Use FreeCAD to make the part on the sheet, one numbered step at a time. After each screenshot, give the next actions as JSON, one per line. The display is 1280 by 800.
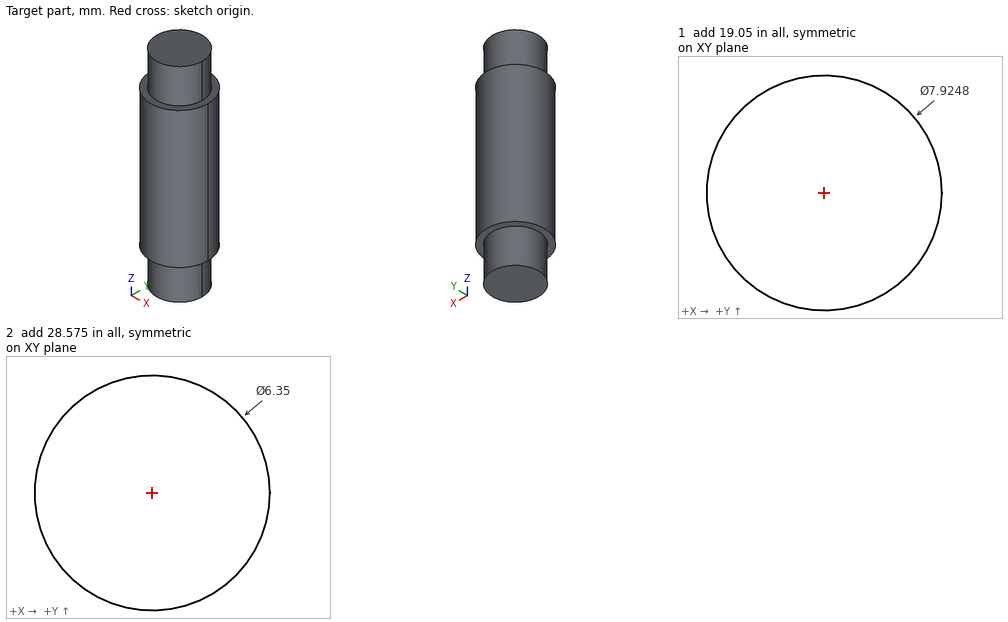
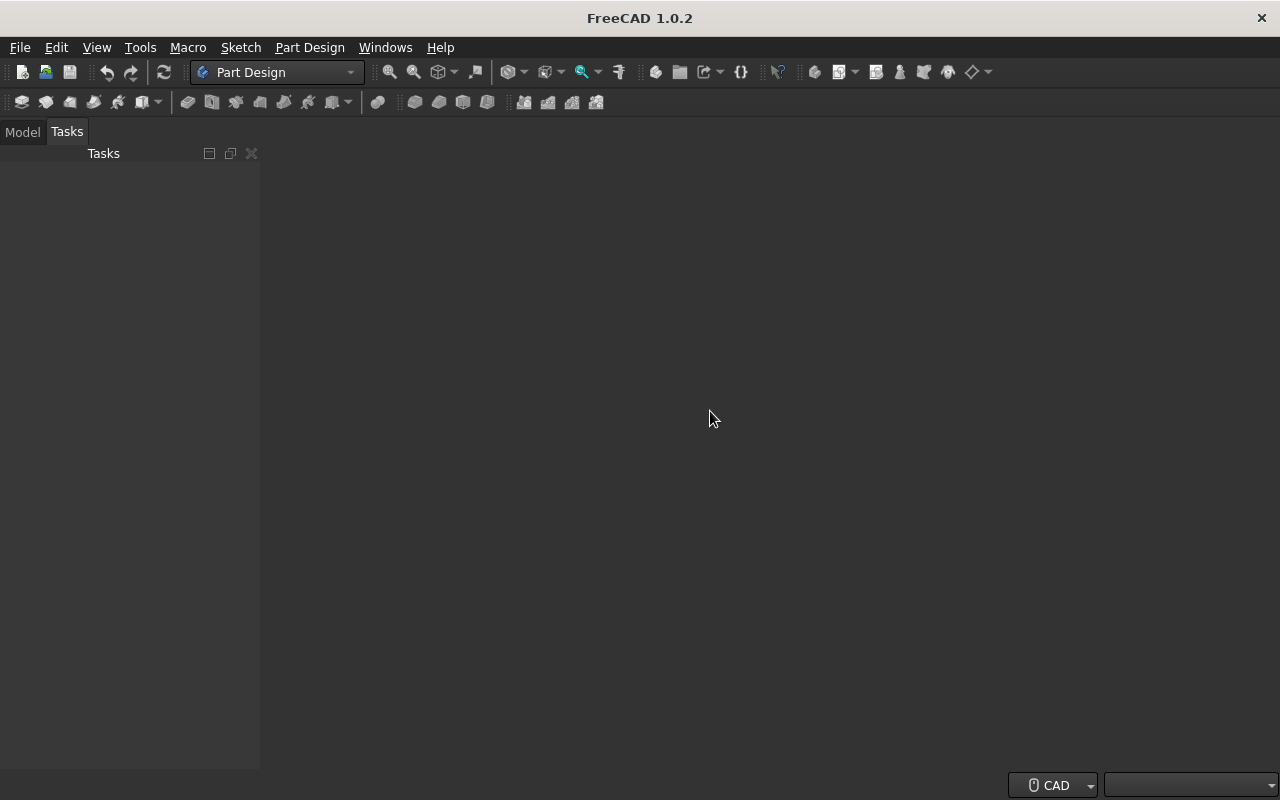
{"action": "left_click", "coordinate": [22, 72]}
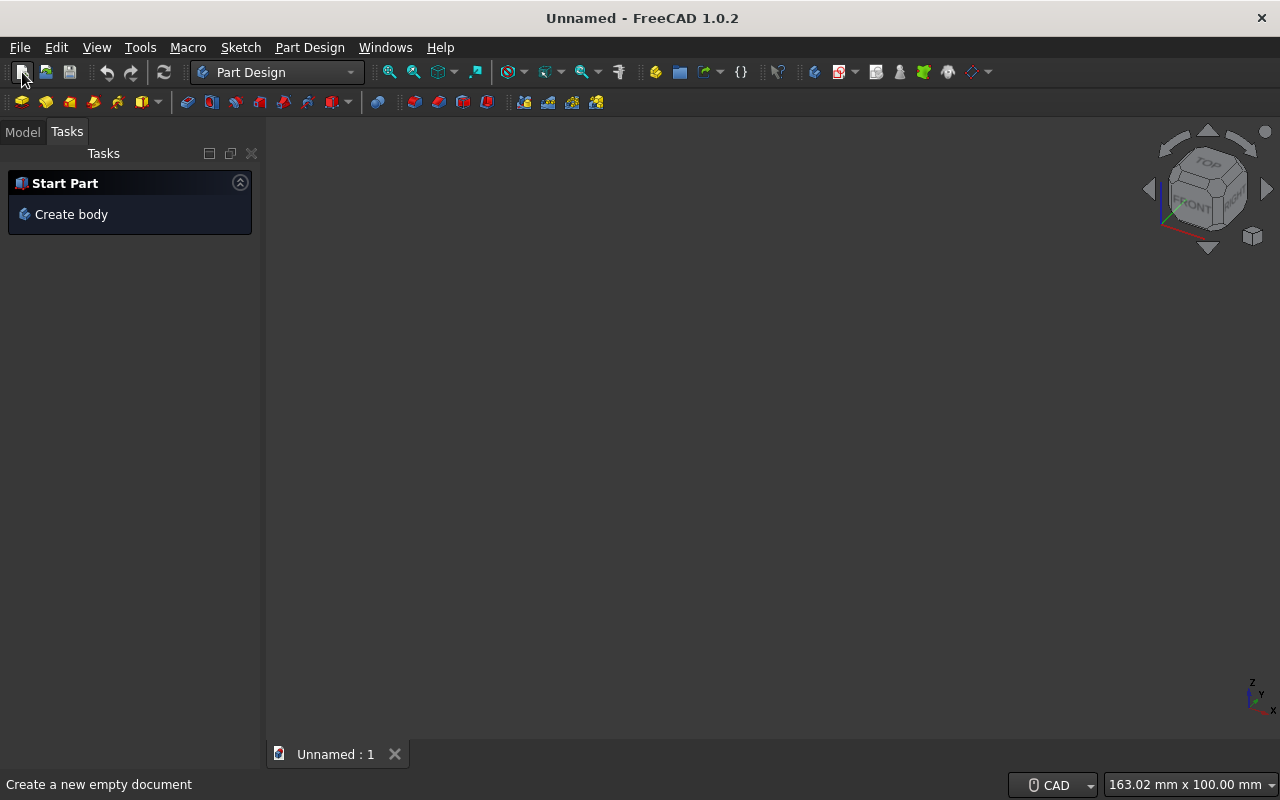
{"action": "left_click", "coordinate": [840, 72]}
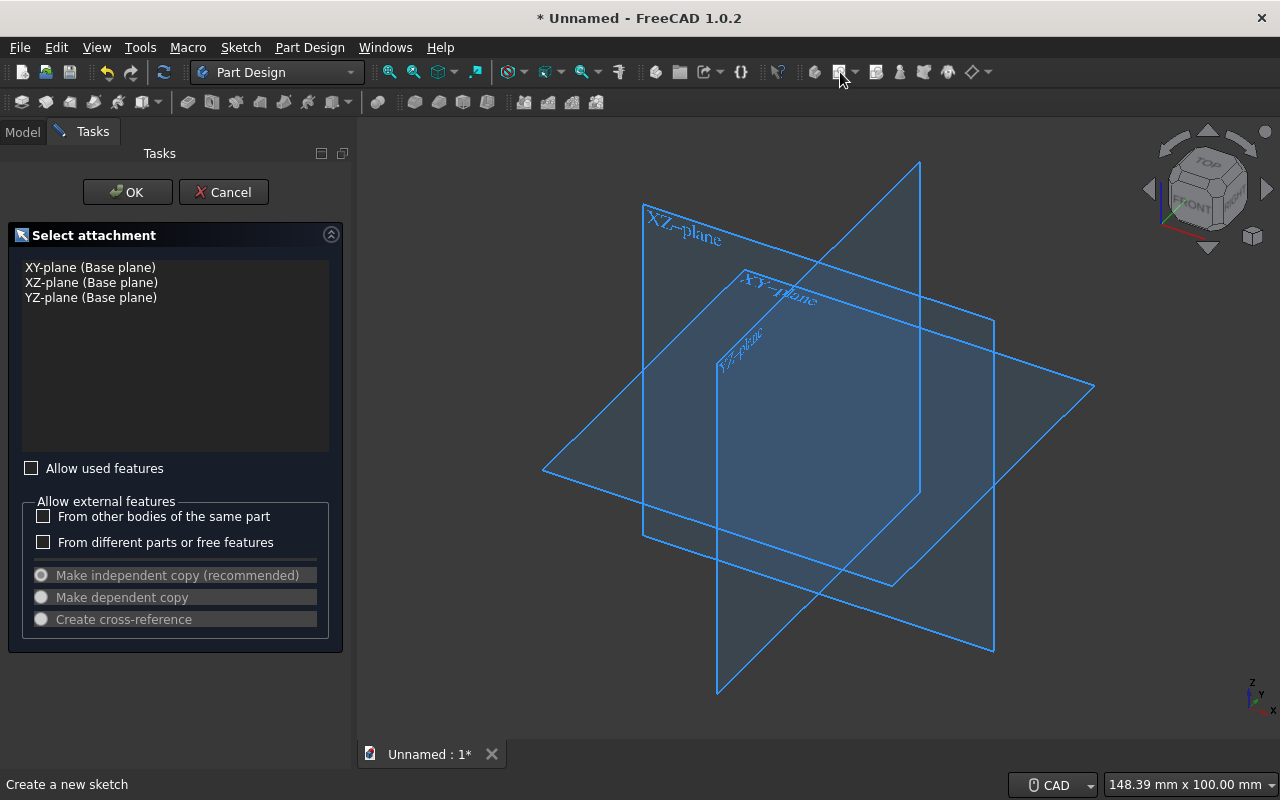
{"action": "left_click", "coordinate": [82, 268]}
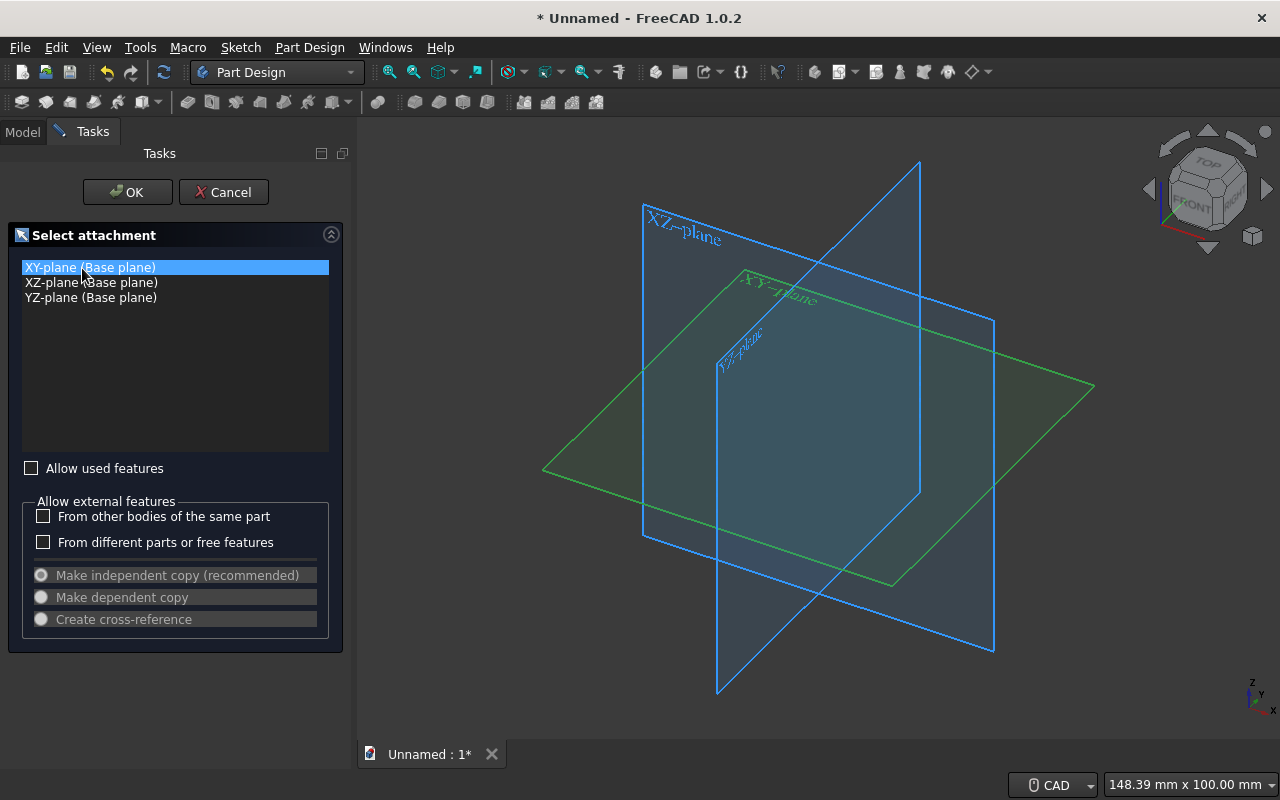
{"action": "left_click", "coordinate": [128, 192]}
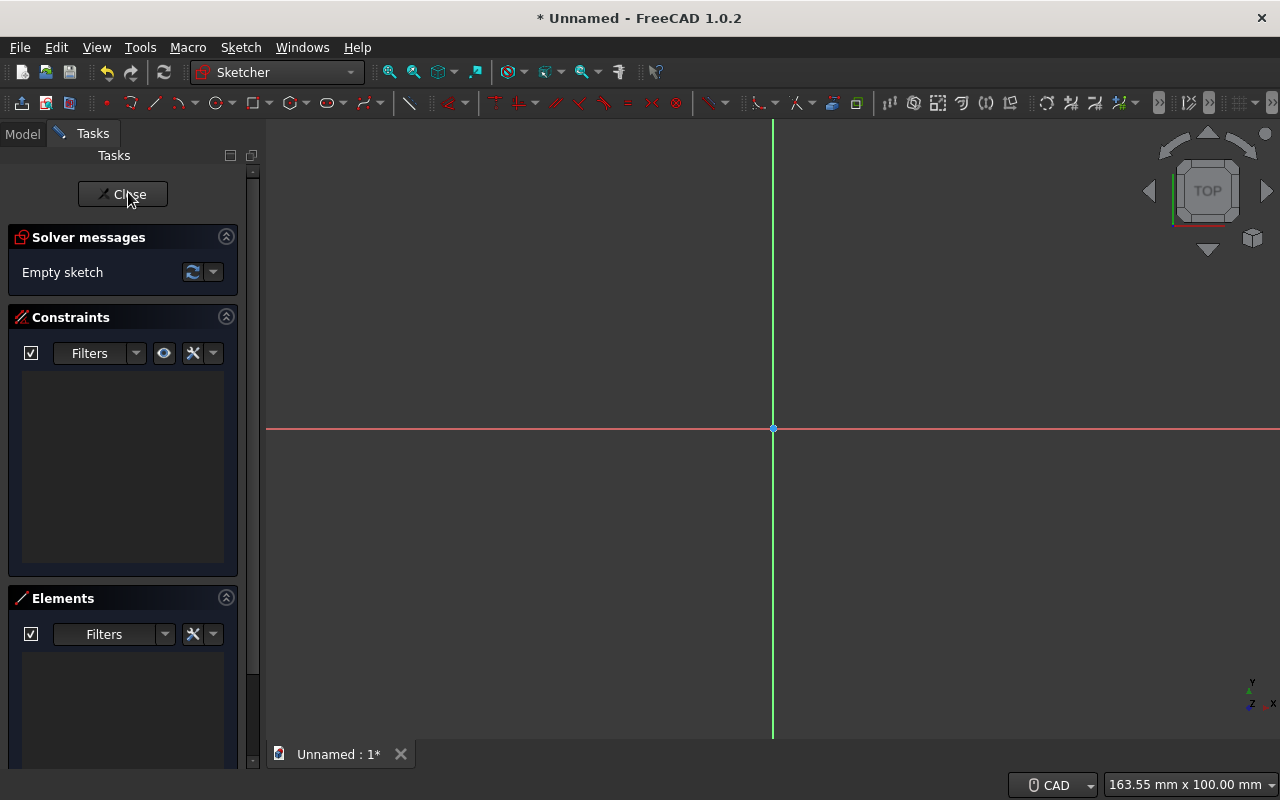
{"action": "scroll", "coordinate": [784, 429], "scroll_direction": "up", "scroll_amount": 10}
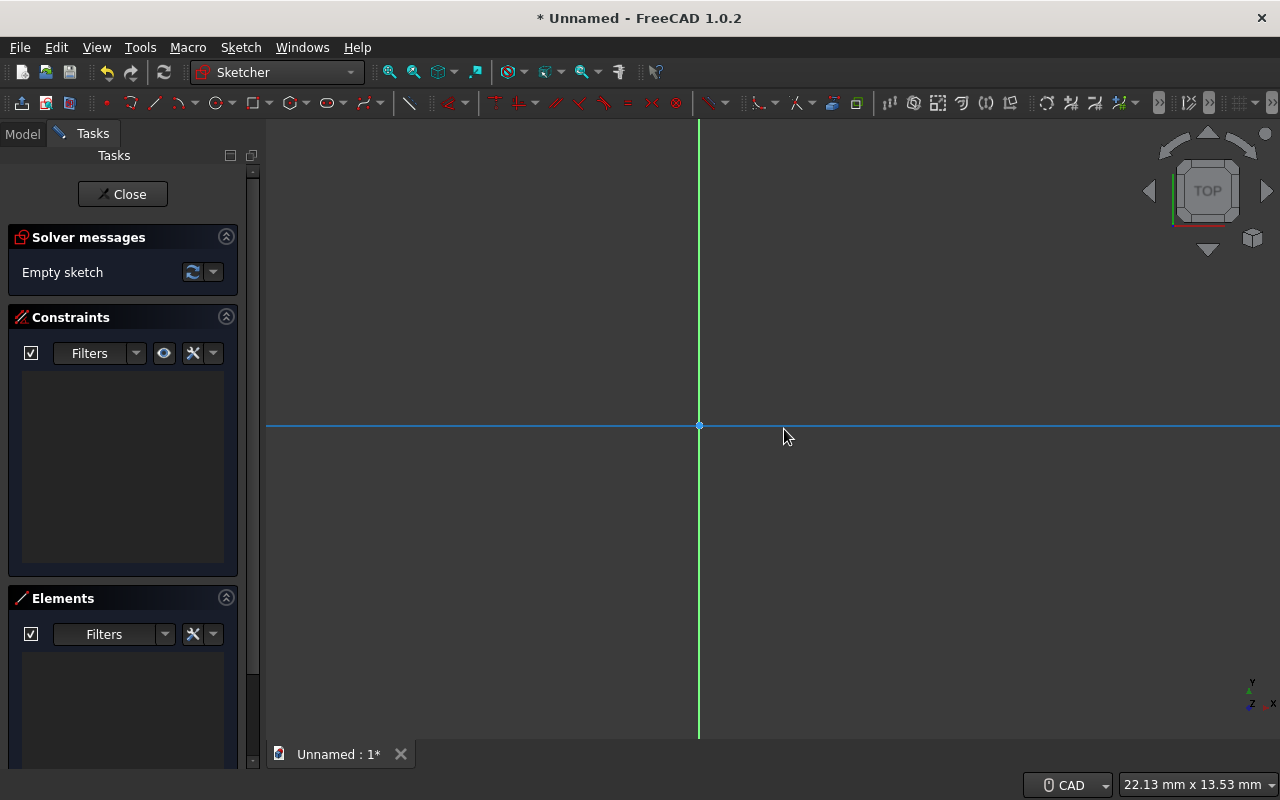
{"action": "left_click", "coordinate": [216, 104]}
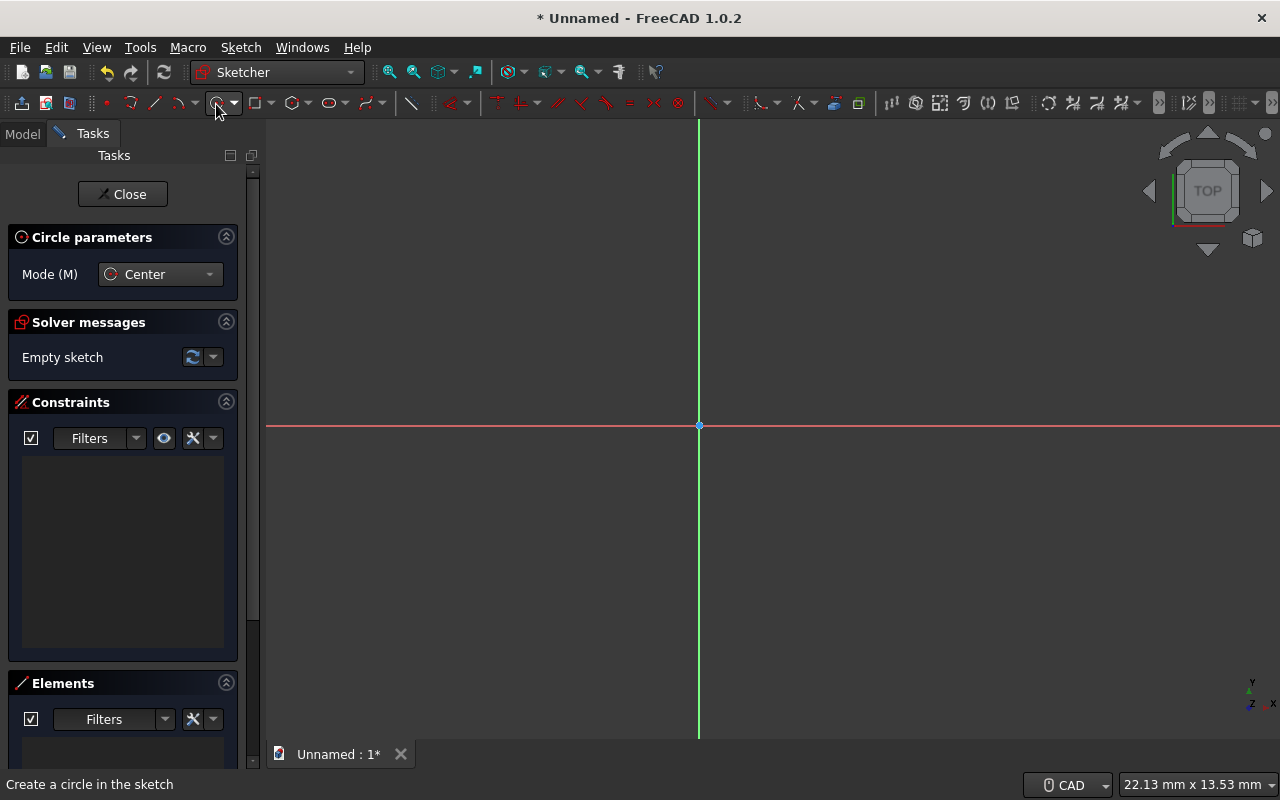
{"action": "left_click", "coordinate": [699, 426]}
{"action": "mouse_move", "coordinate": [828, 297]}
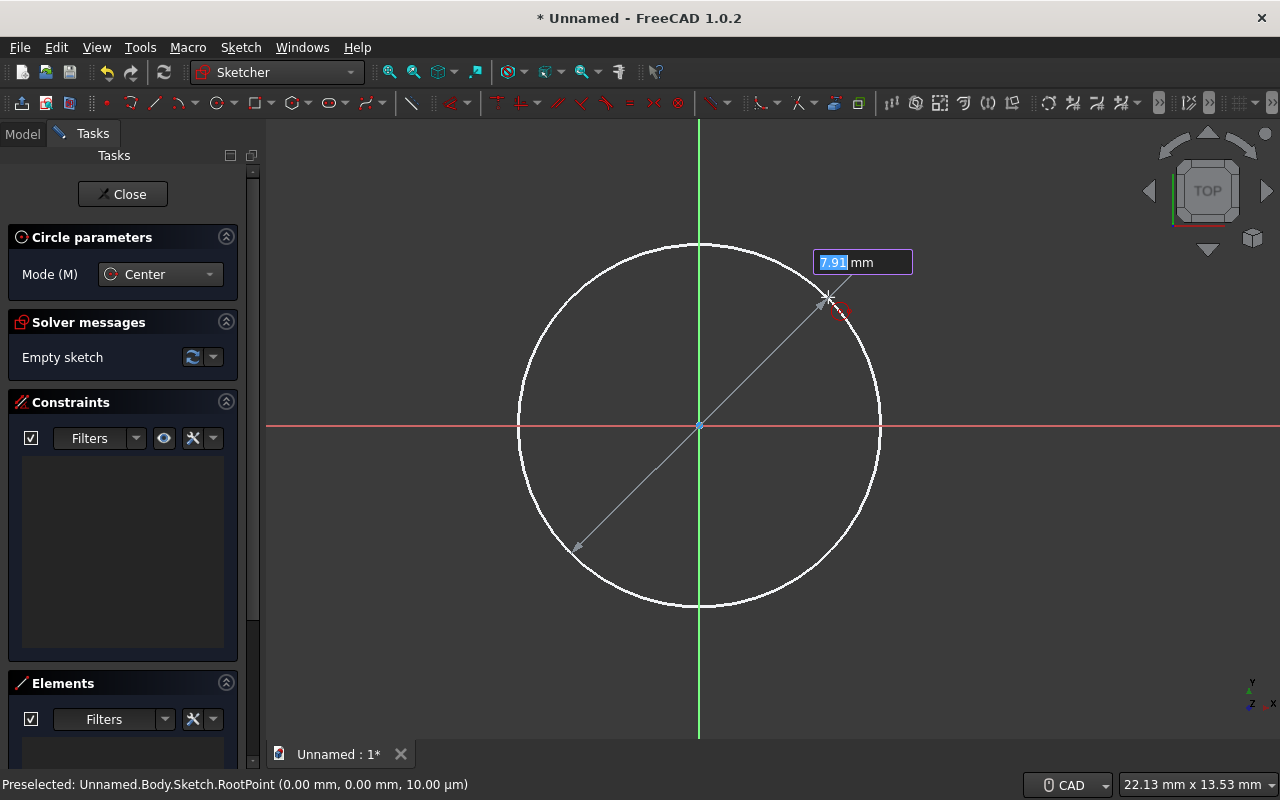
{"action": "type", "text": "7.9248"}
{"action": "key", "text": "Return"}
{"action": "key", "text": "Escape"}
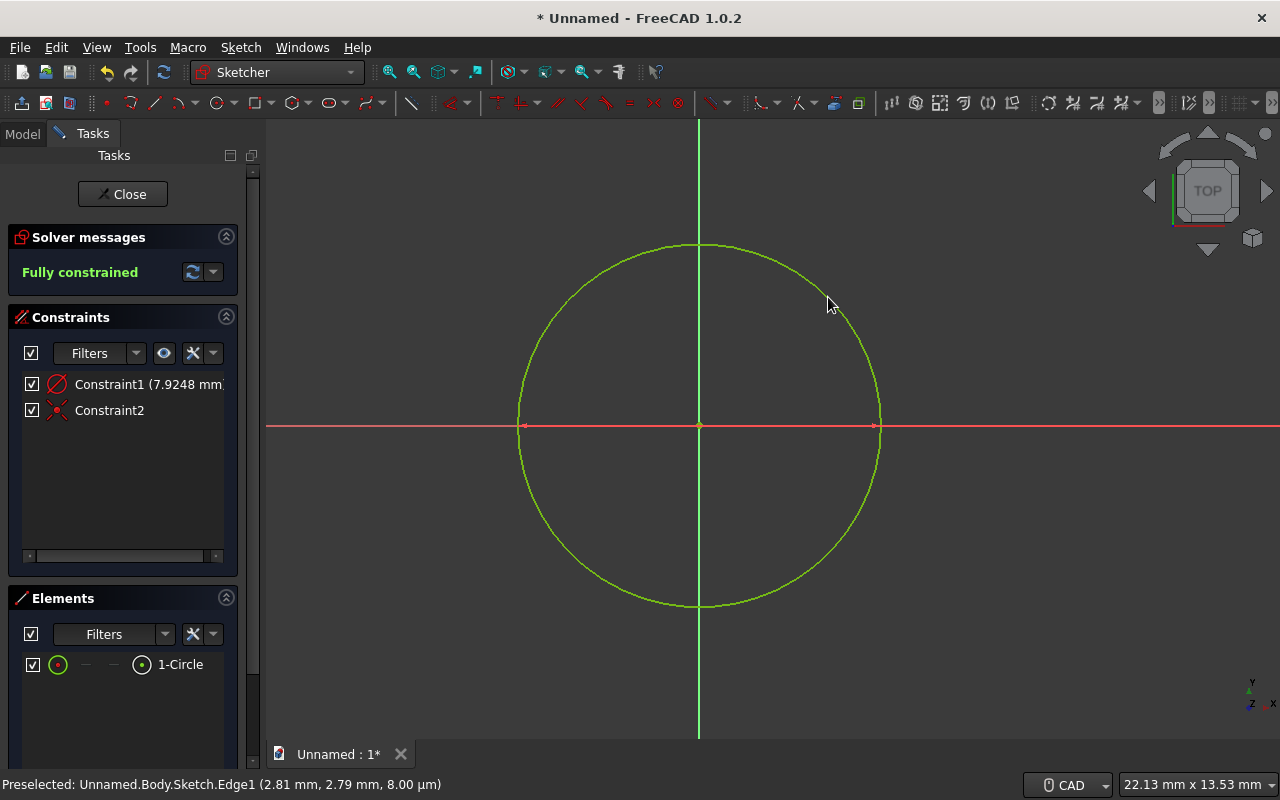
{"action": "left_click", "coordinate": [123, 194]}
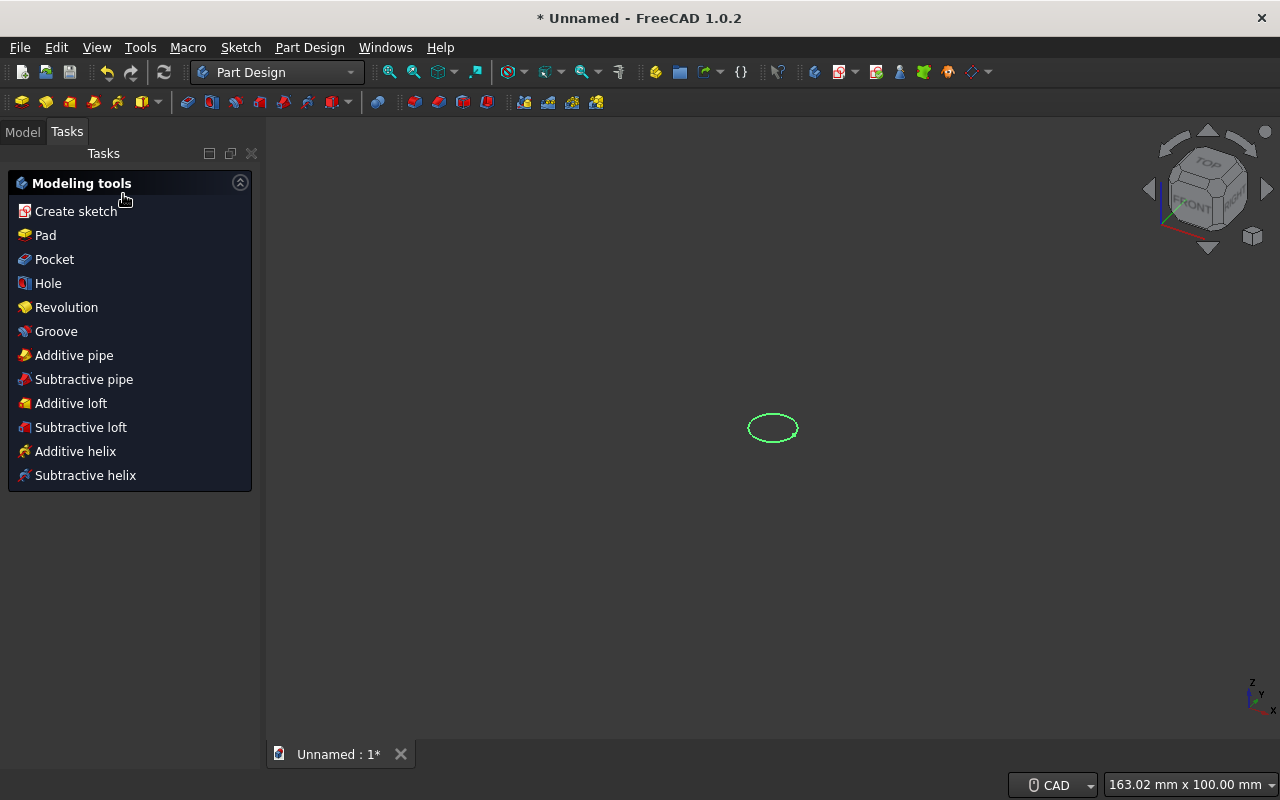
{"action": "left_click", "coordinate": [22, 102]}